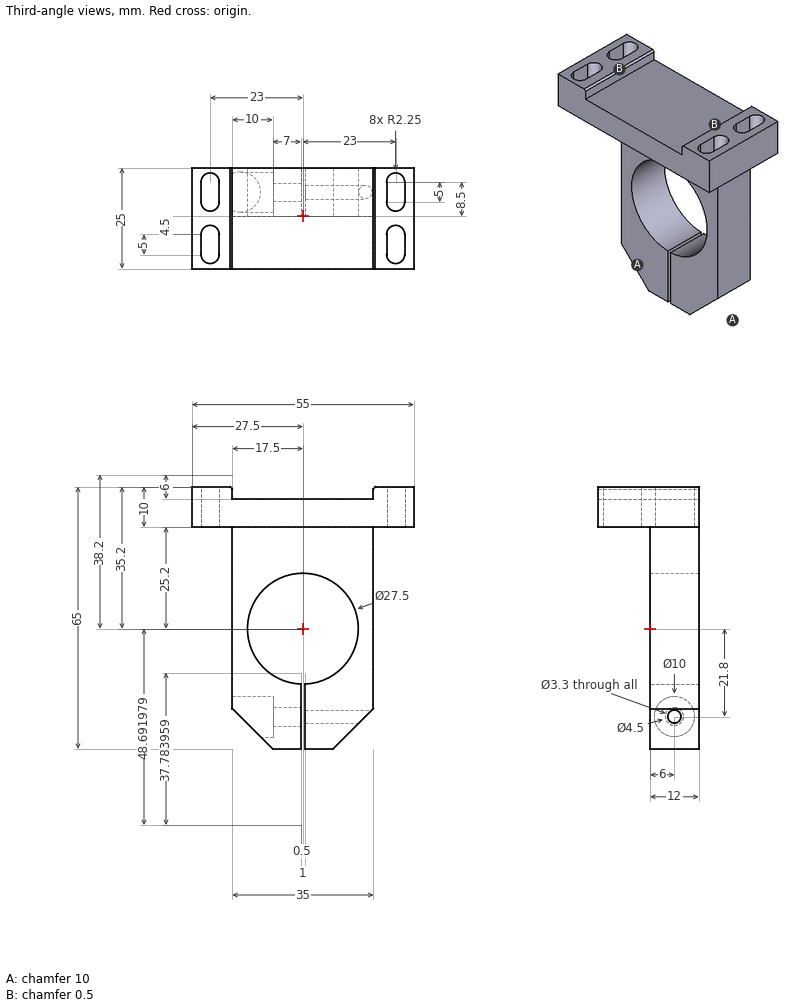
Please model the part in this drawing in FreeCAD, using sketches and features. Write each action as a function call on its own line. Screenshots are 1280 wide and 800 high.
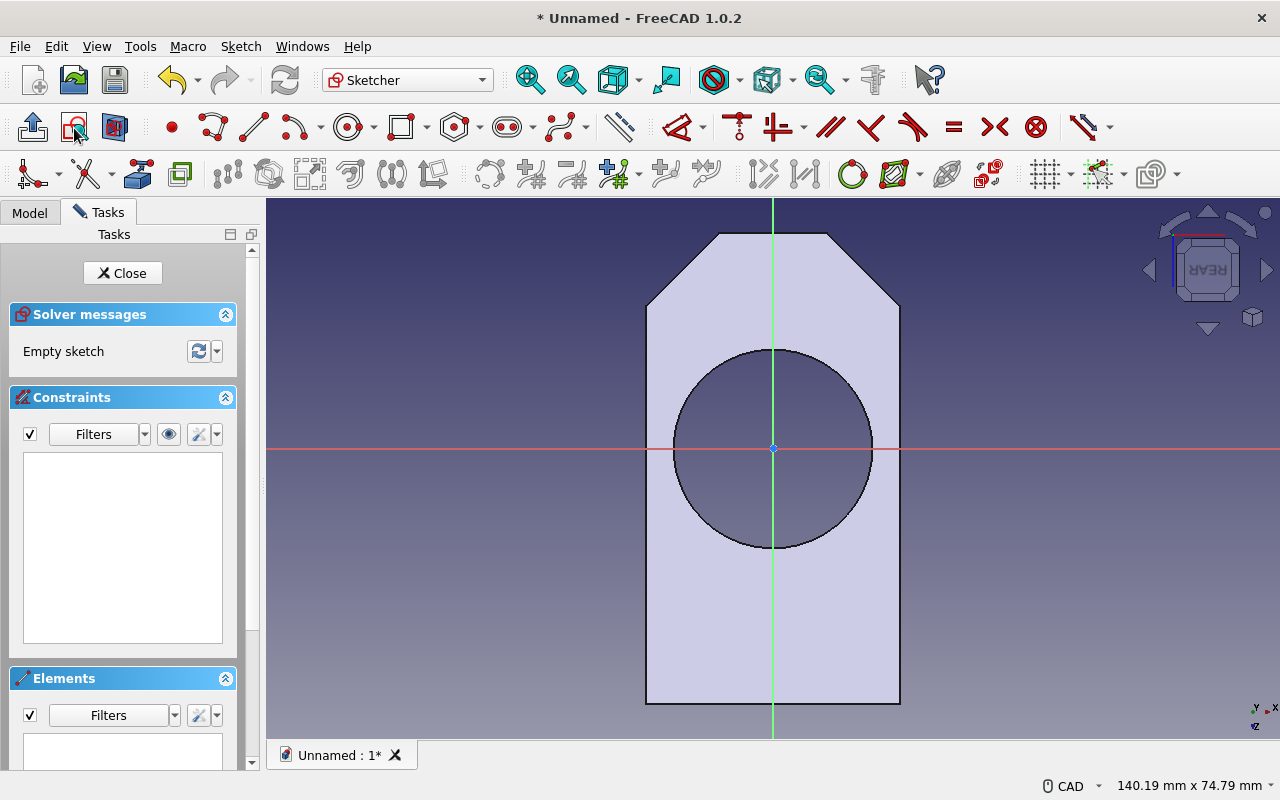
scroll(395, 226, down, 1)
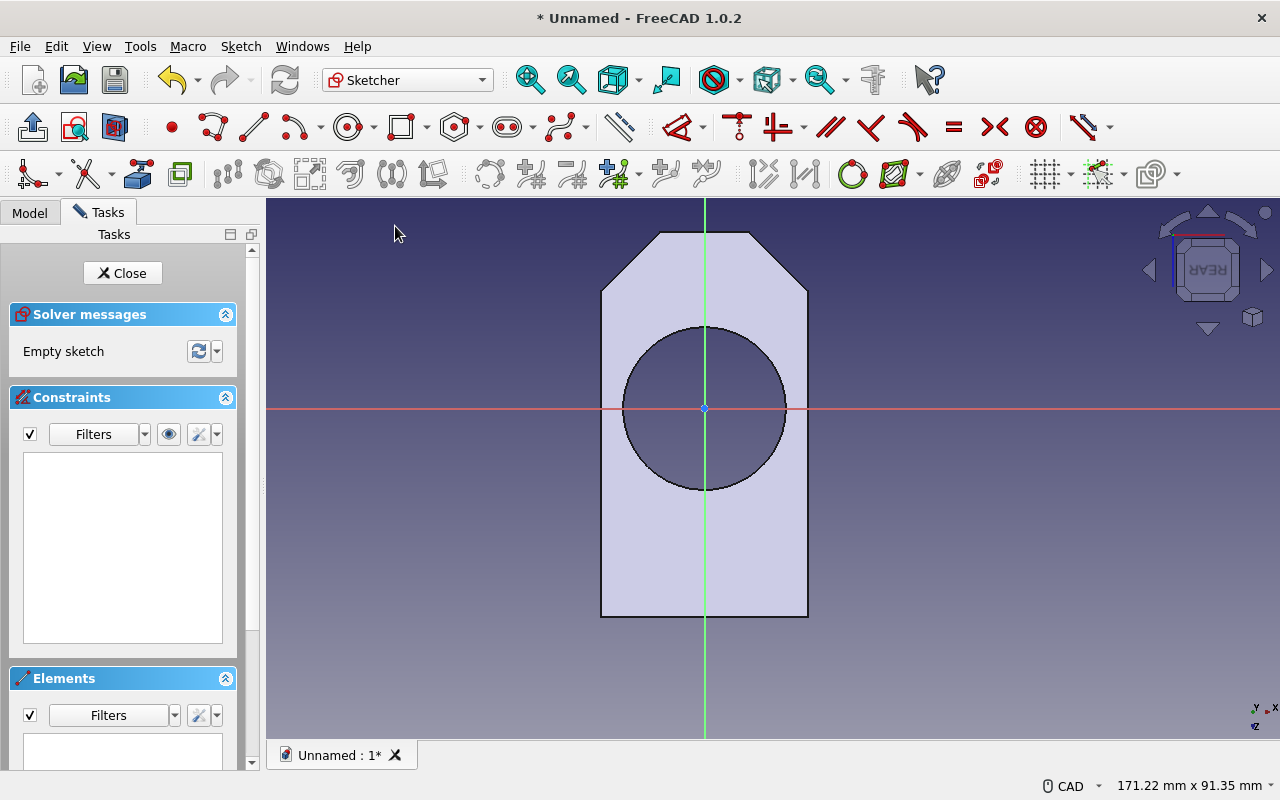
scroll(705, 603, up, 2)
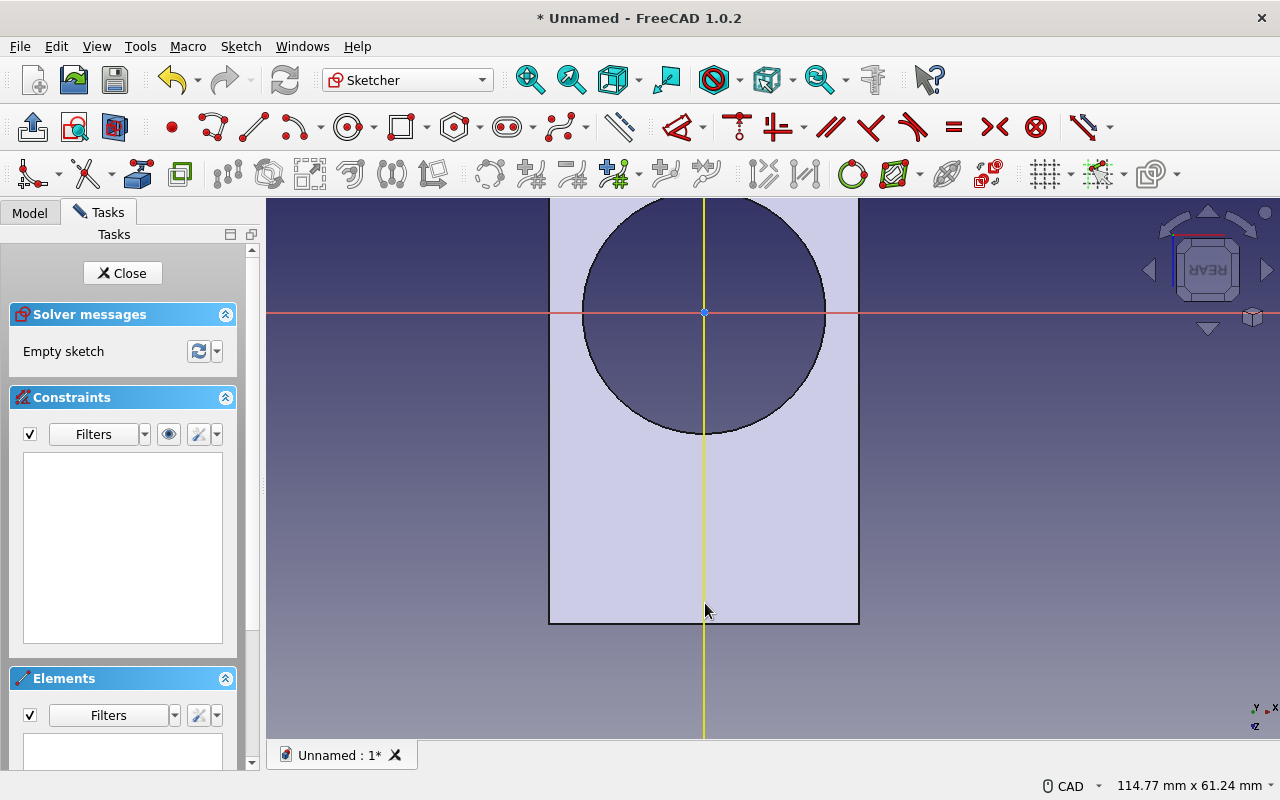
click(400, 128)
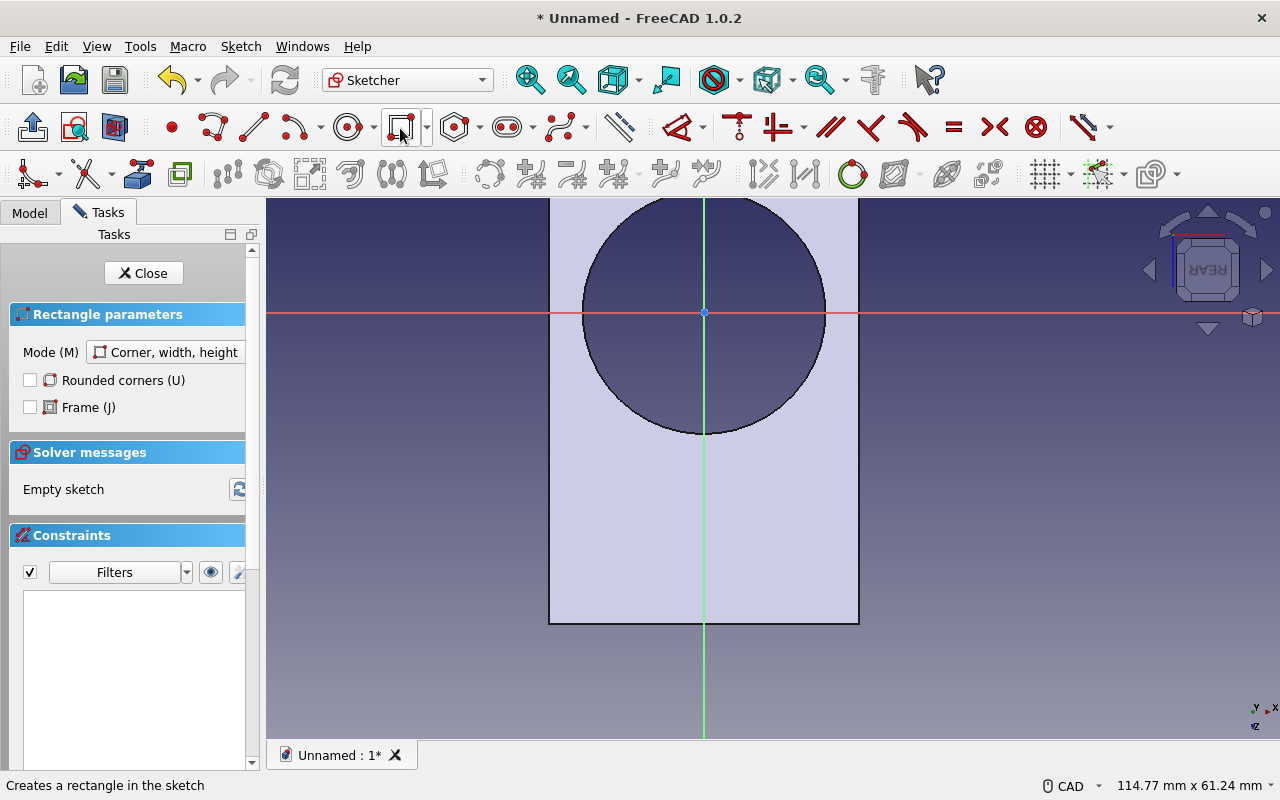
click(461, 535)
click(947, 624)
key(Escape)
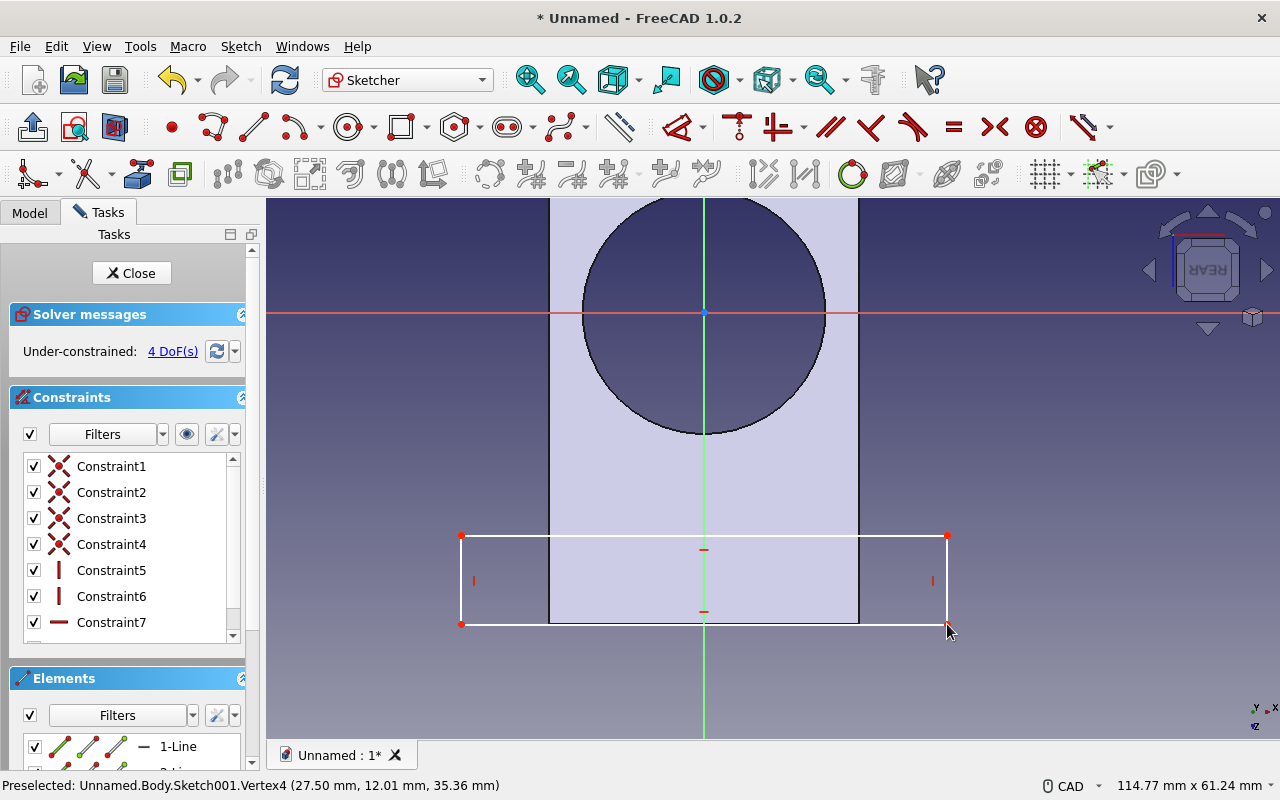
click(676, 128)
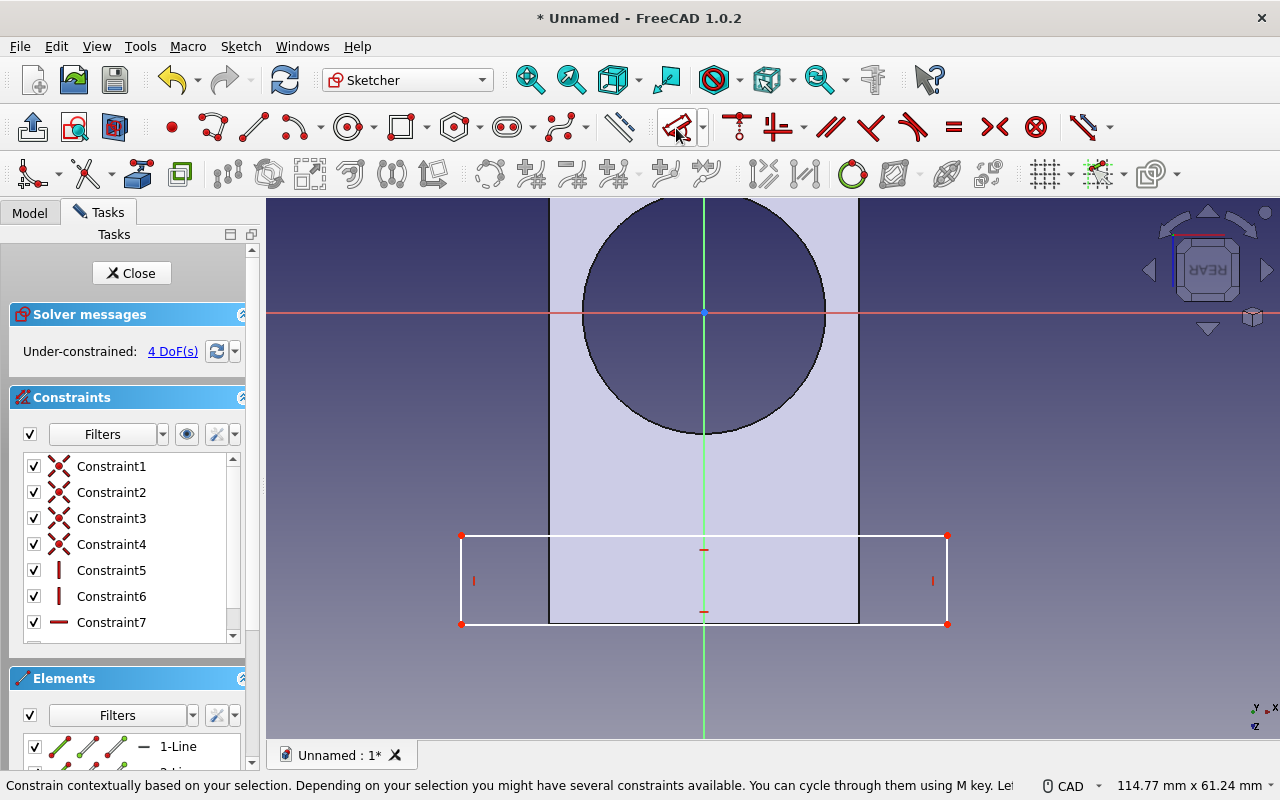
click(461, 563)
click(427, 580)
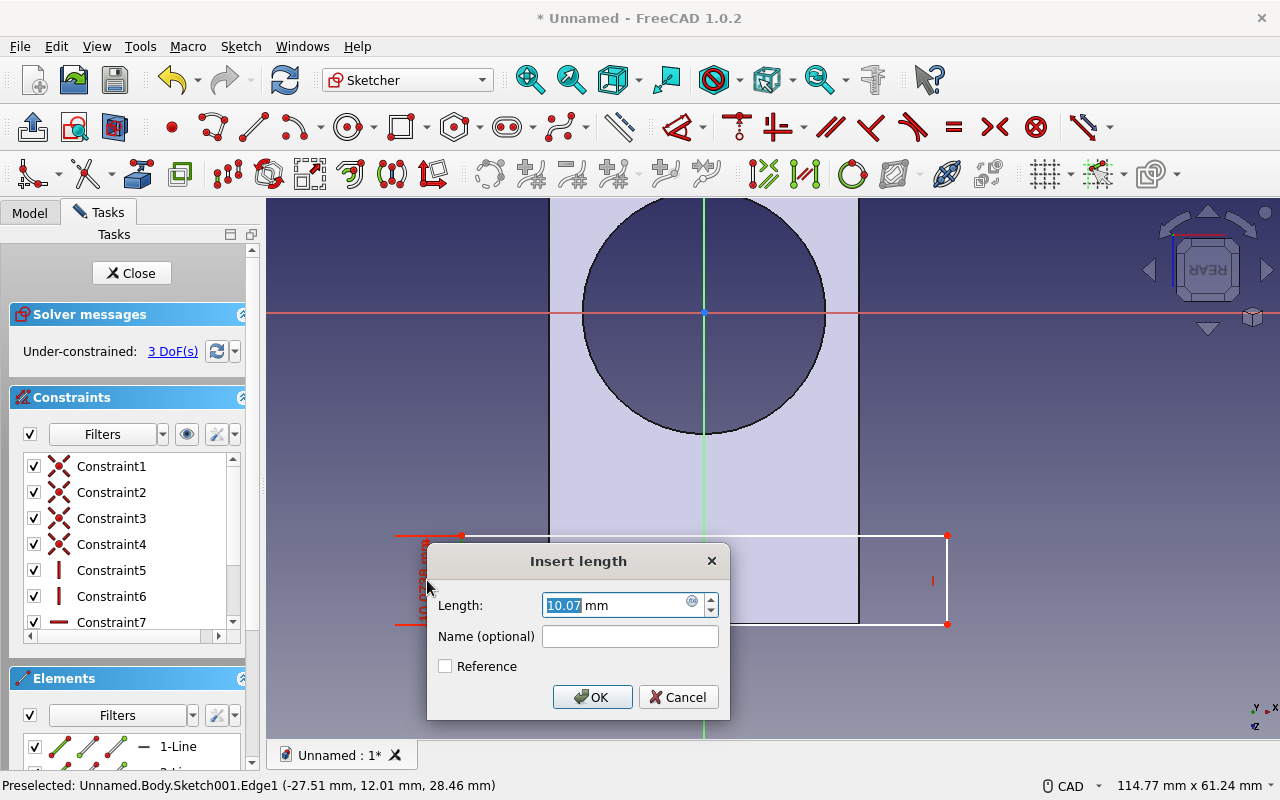
text(10)
key(Return)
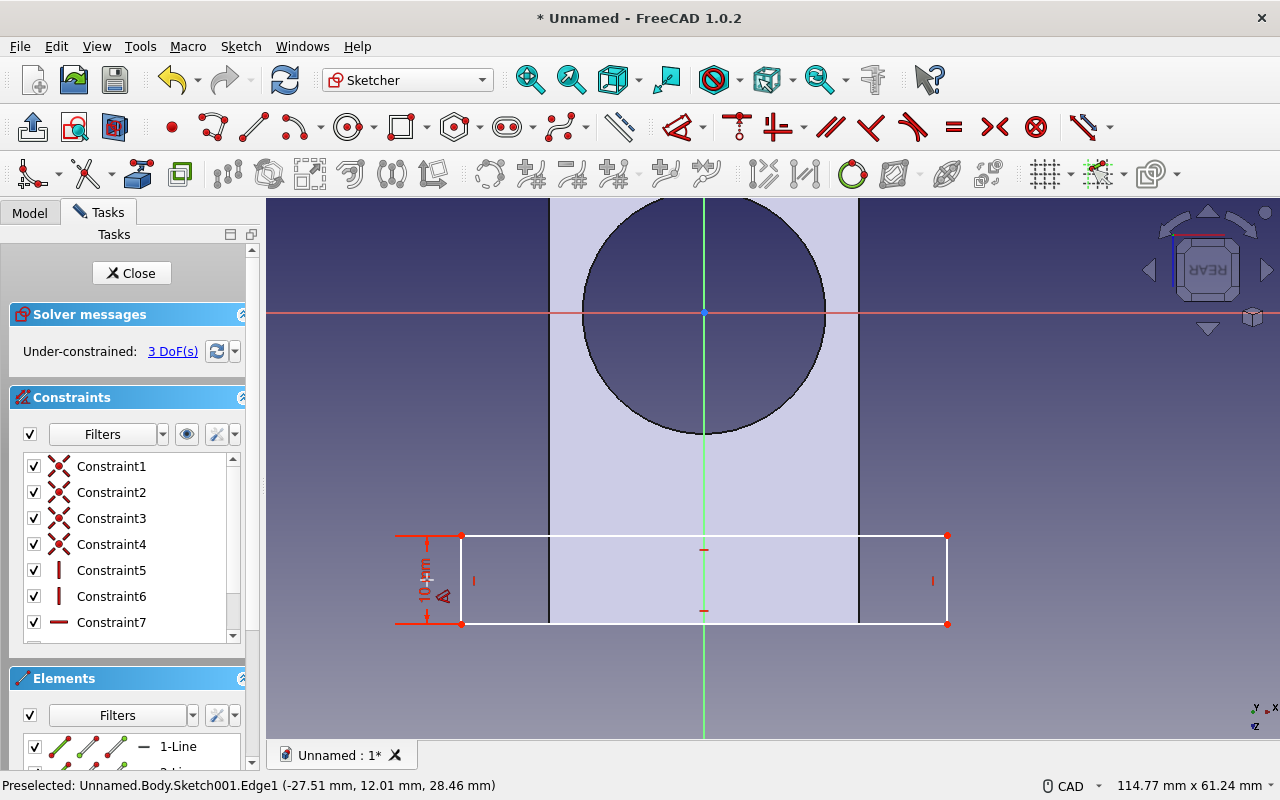
click(607, 624)
click(592, 658)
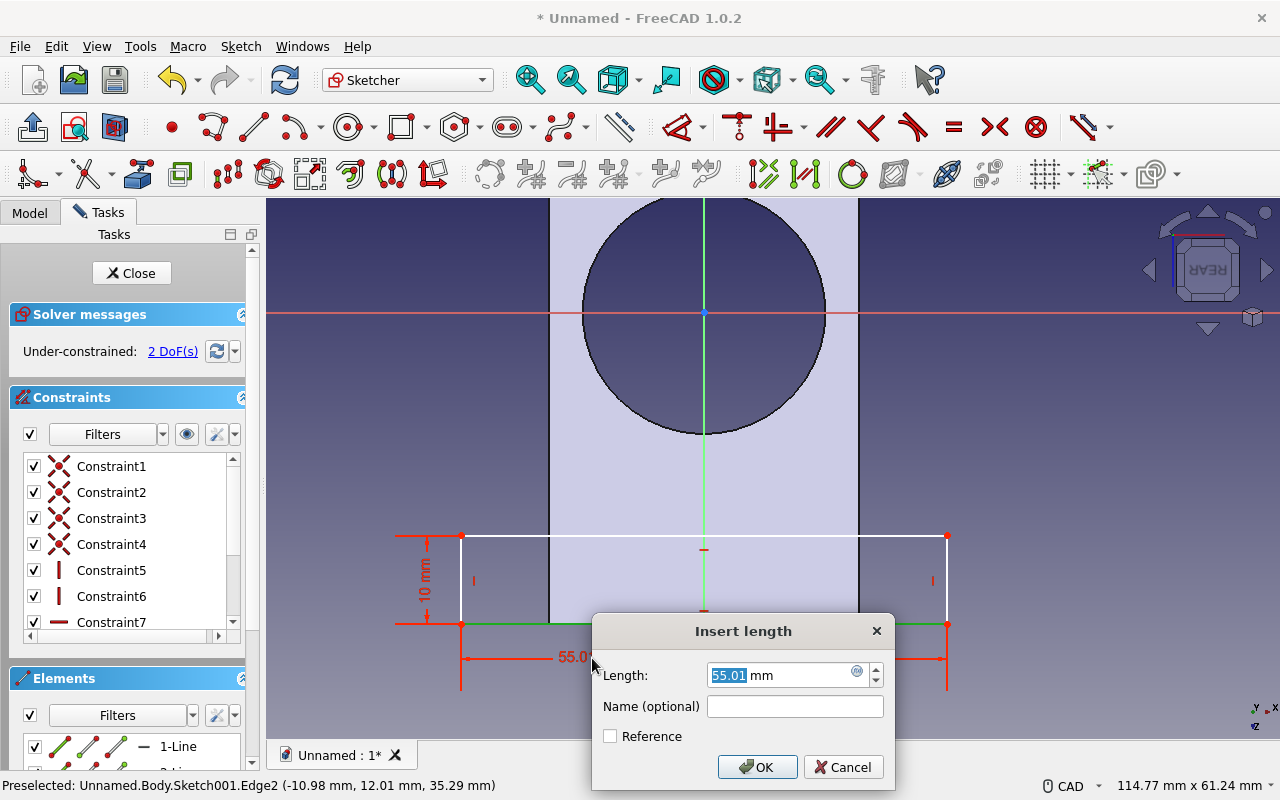
text(55)
key(Return)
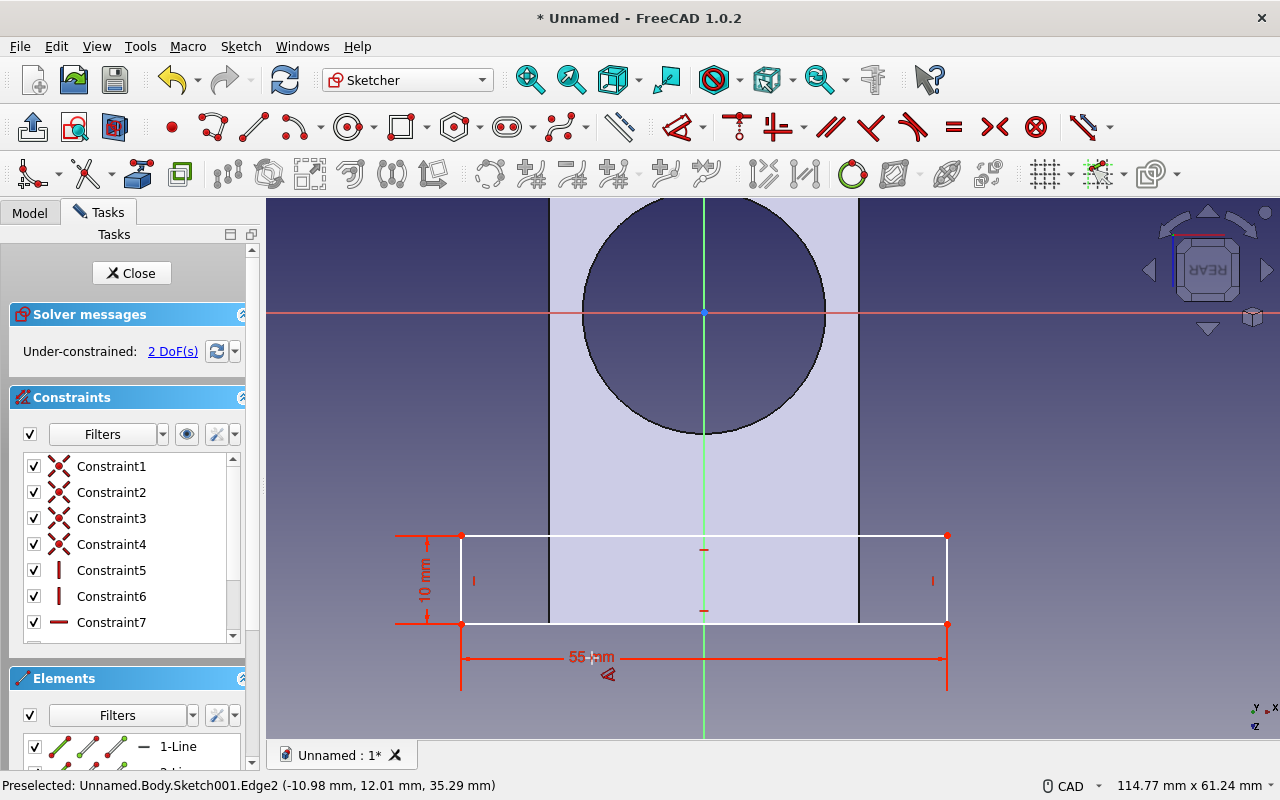
click(461, 536)
click(583, 279)